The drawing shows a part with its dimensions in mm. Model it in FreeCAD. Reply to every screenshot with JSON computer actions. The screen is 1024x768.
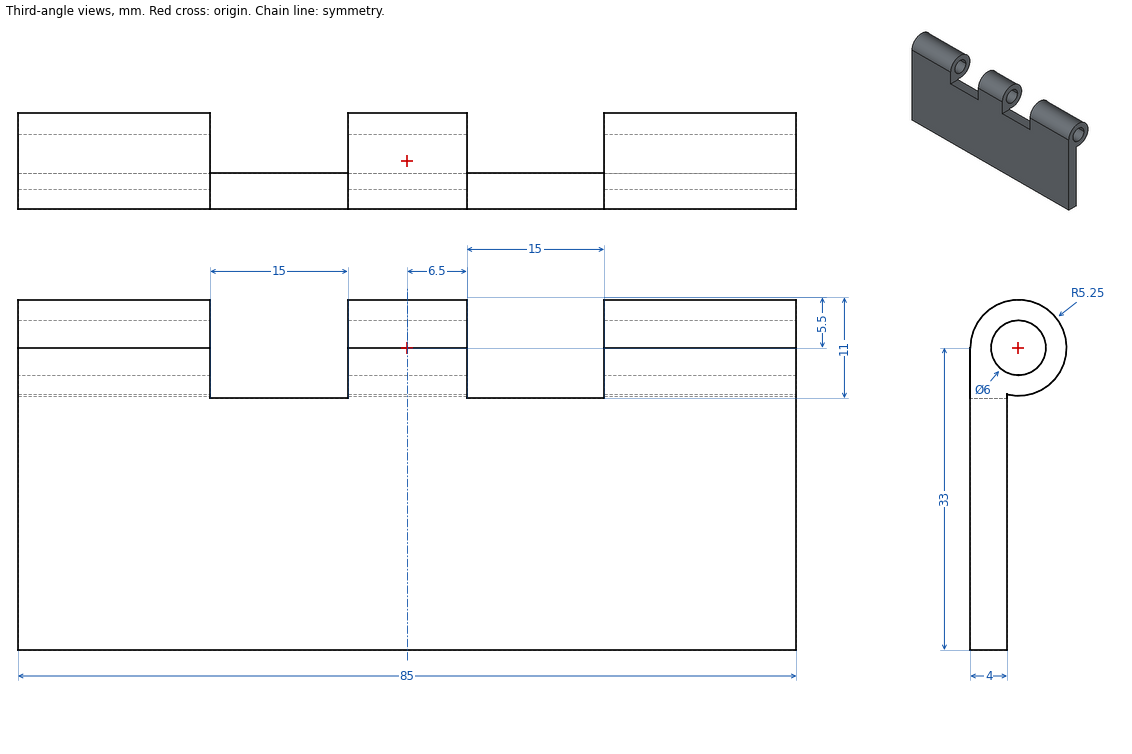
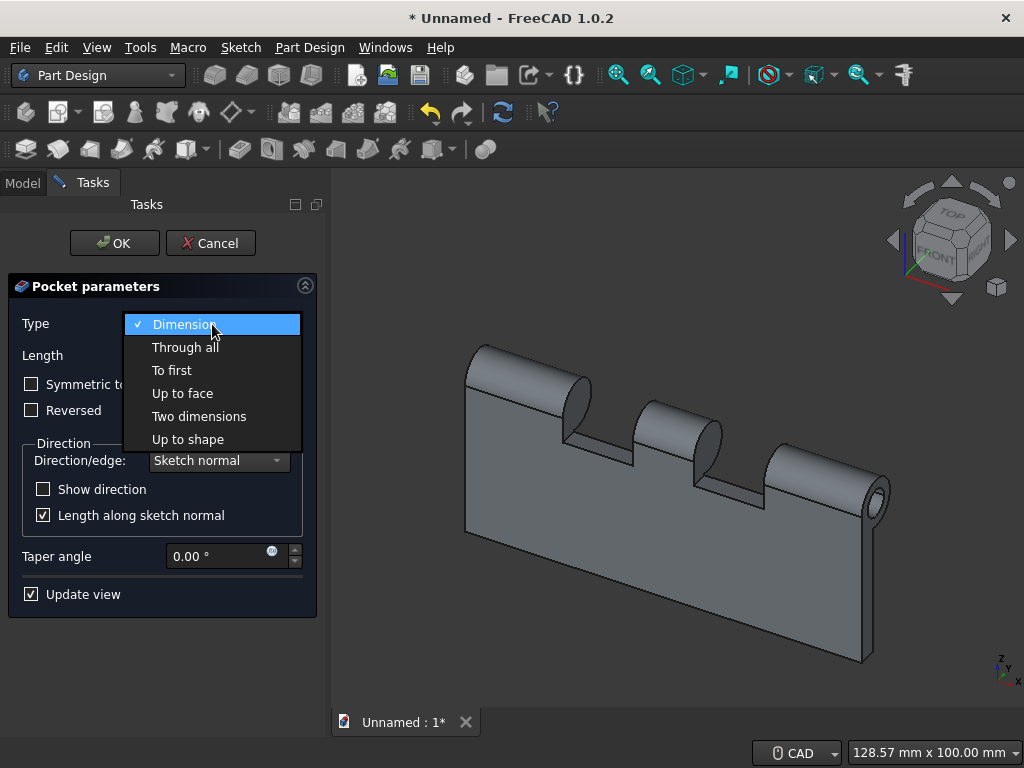
{"action": "left_click", "coordinate": [212, 348]}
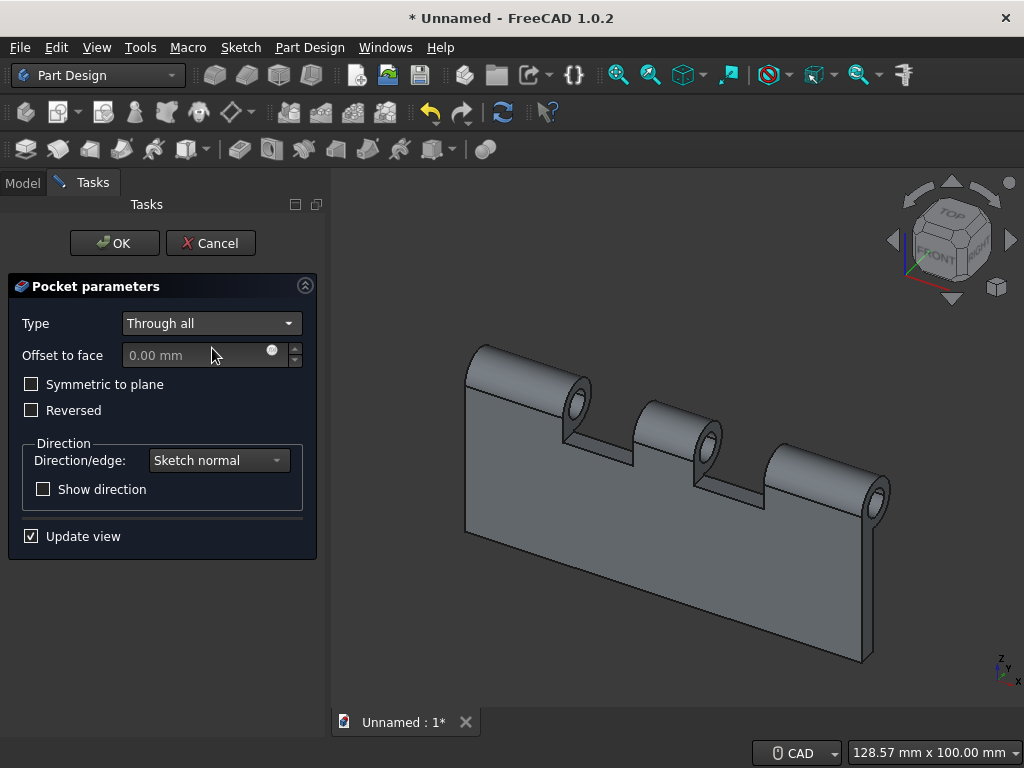
{"action": "left_click", "coordinate": [115, 243]}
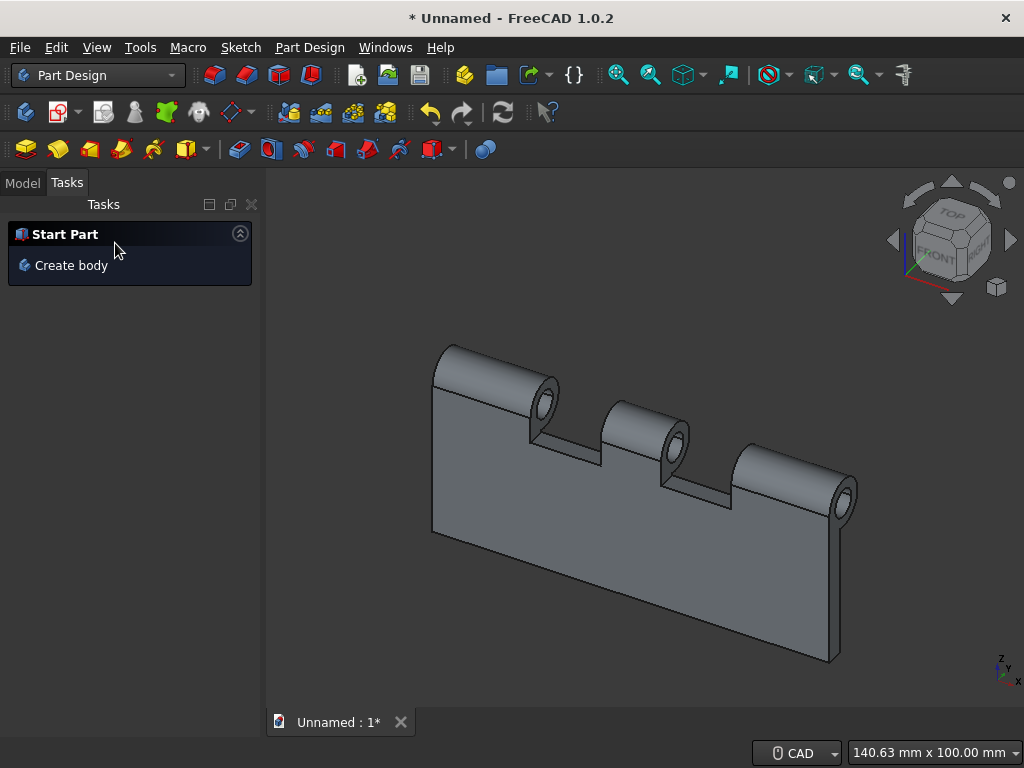
{"action": "key", "text": "0"}